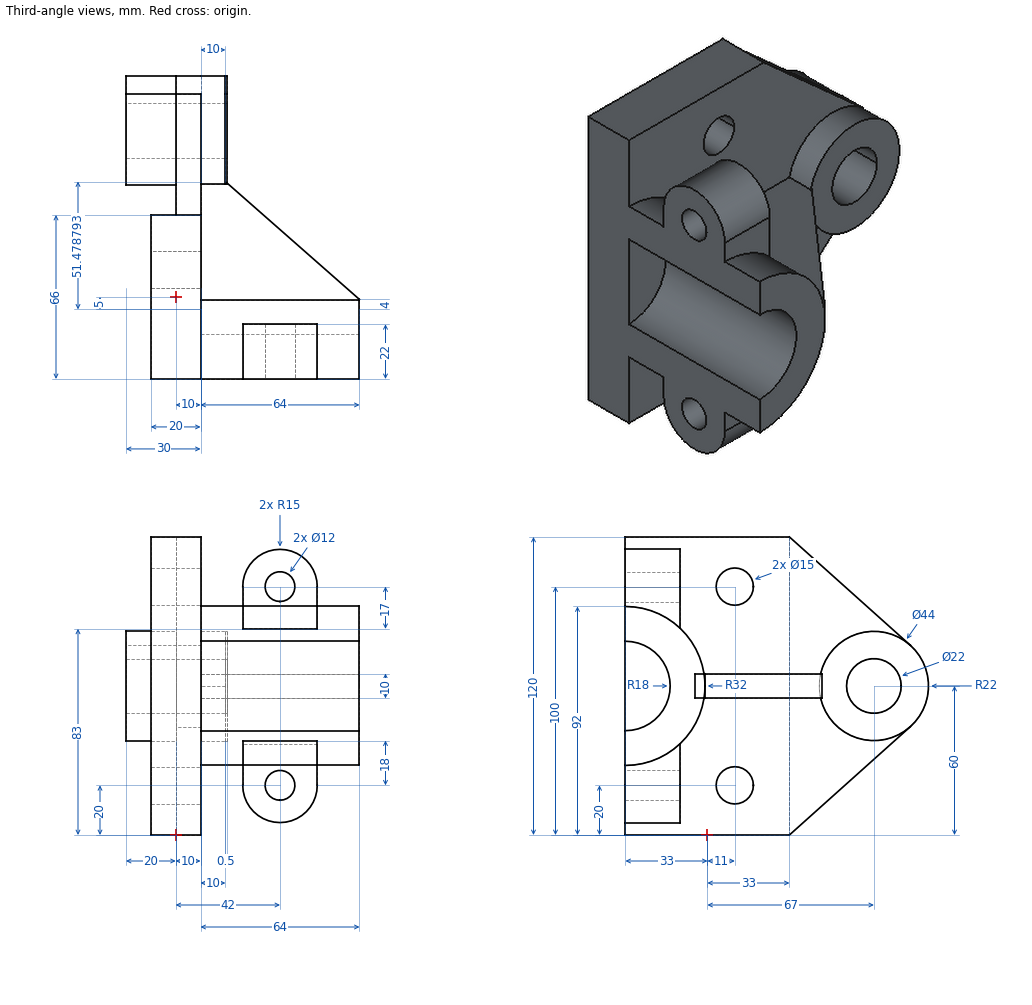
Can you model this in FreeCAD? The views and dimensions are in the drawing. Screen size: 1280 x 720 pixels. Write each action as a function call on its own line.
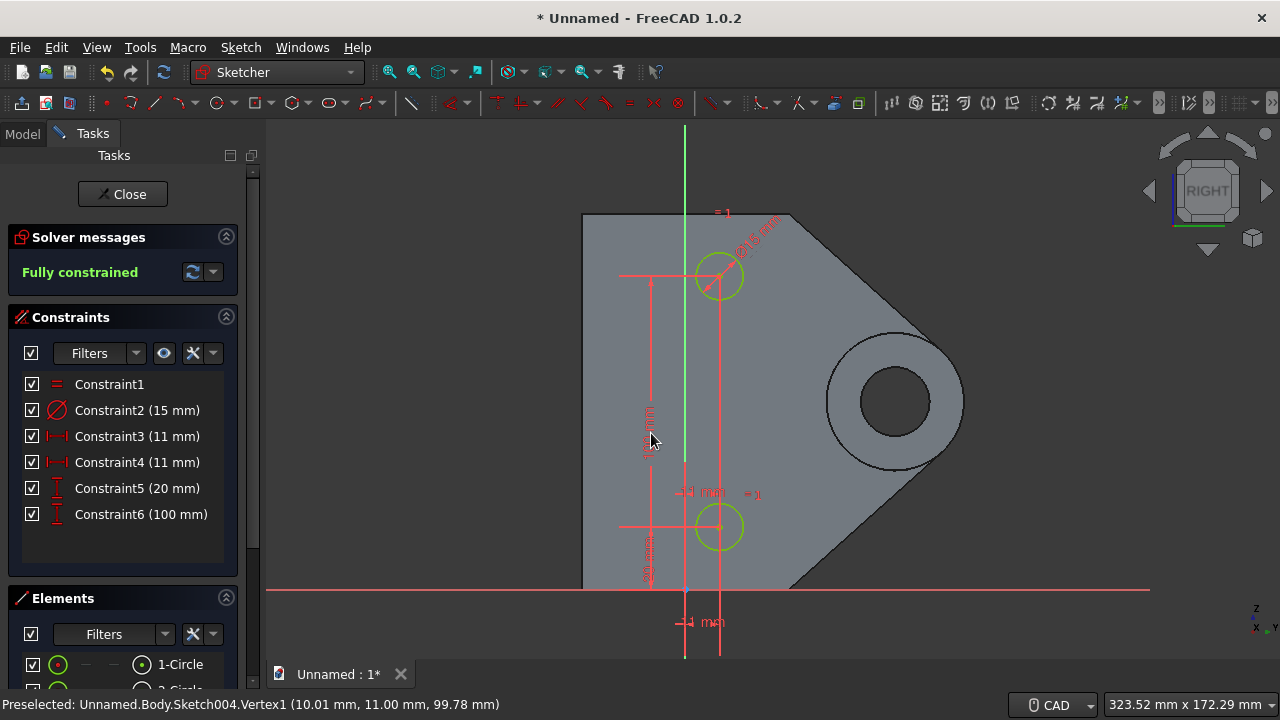
click(123, 194)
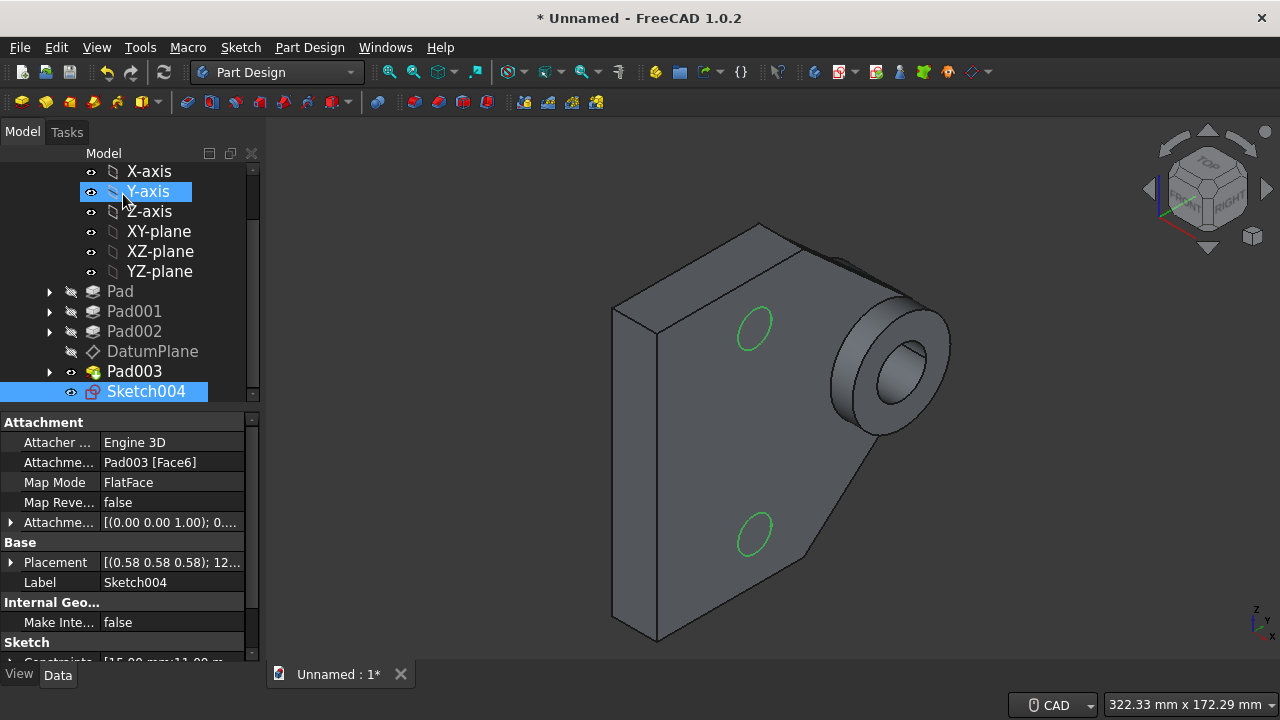
click(188, 102)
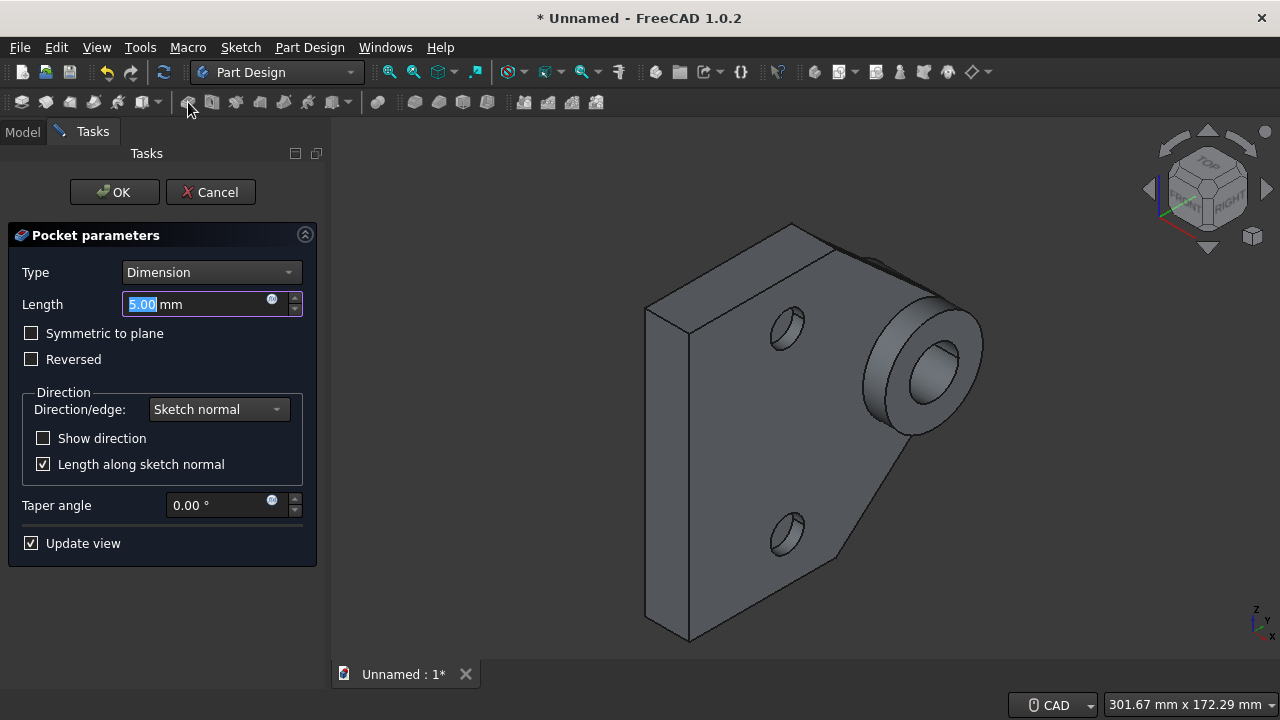
text(30)
key(Tab)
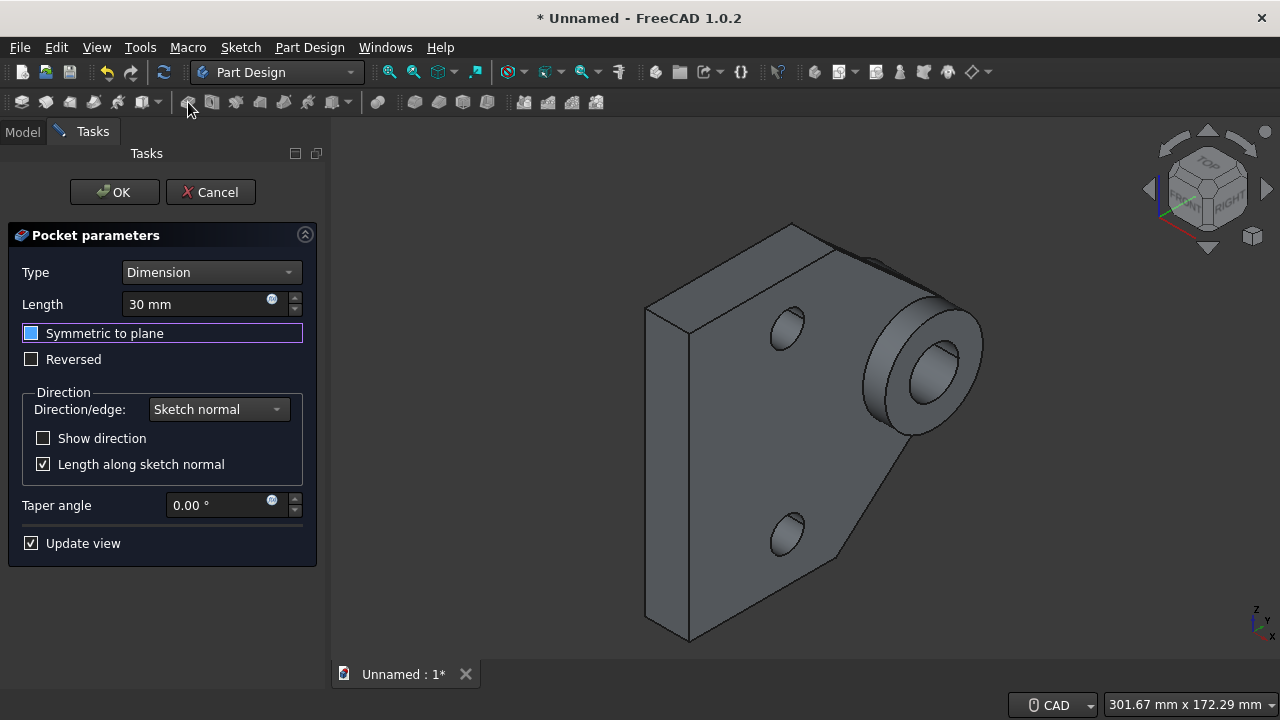
click(115, 192)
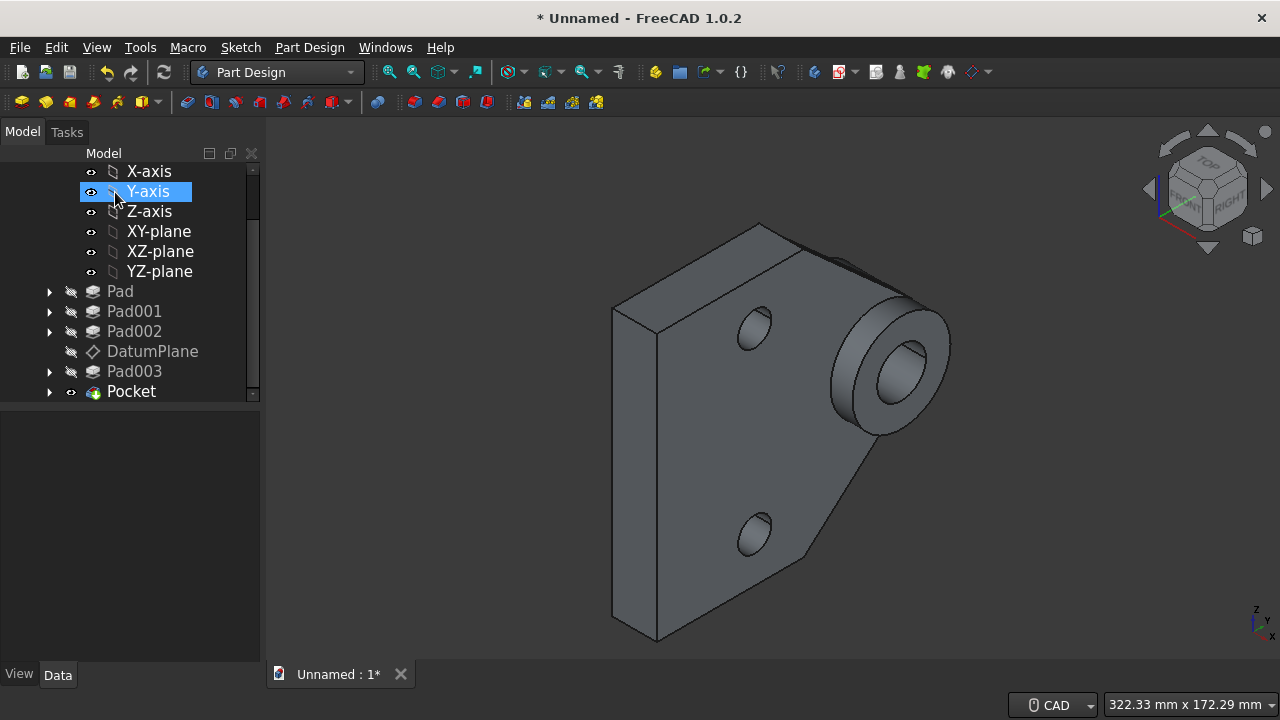
click(748, 434)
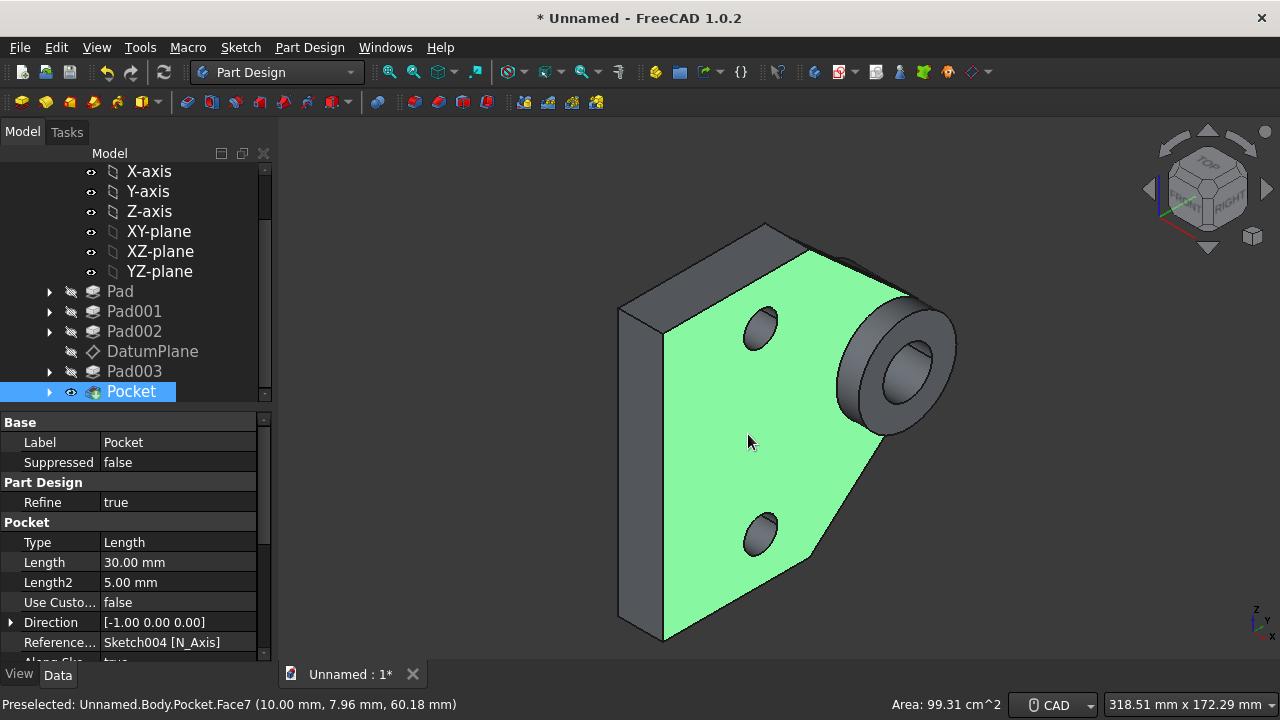
click(840, 72)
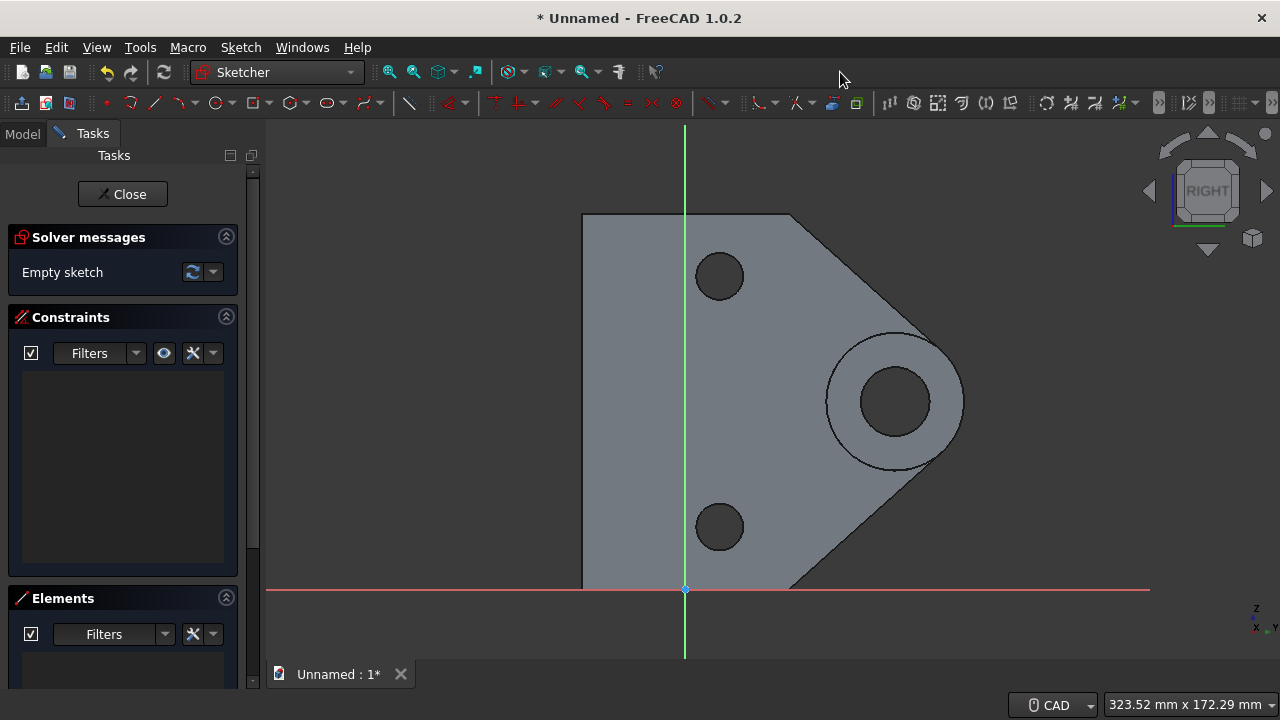
click(70, 104)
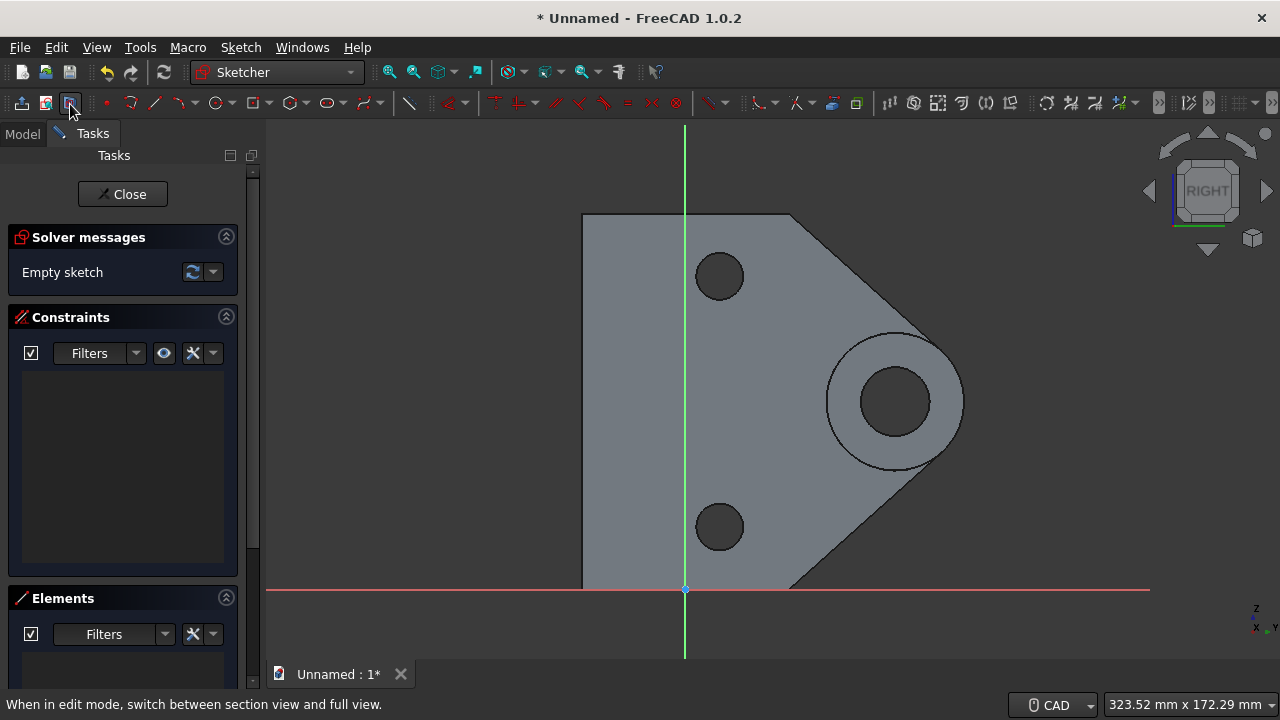
click(156, 104)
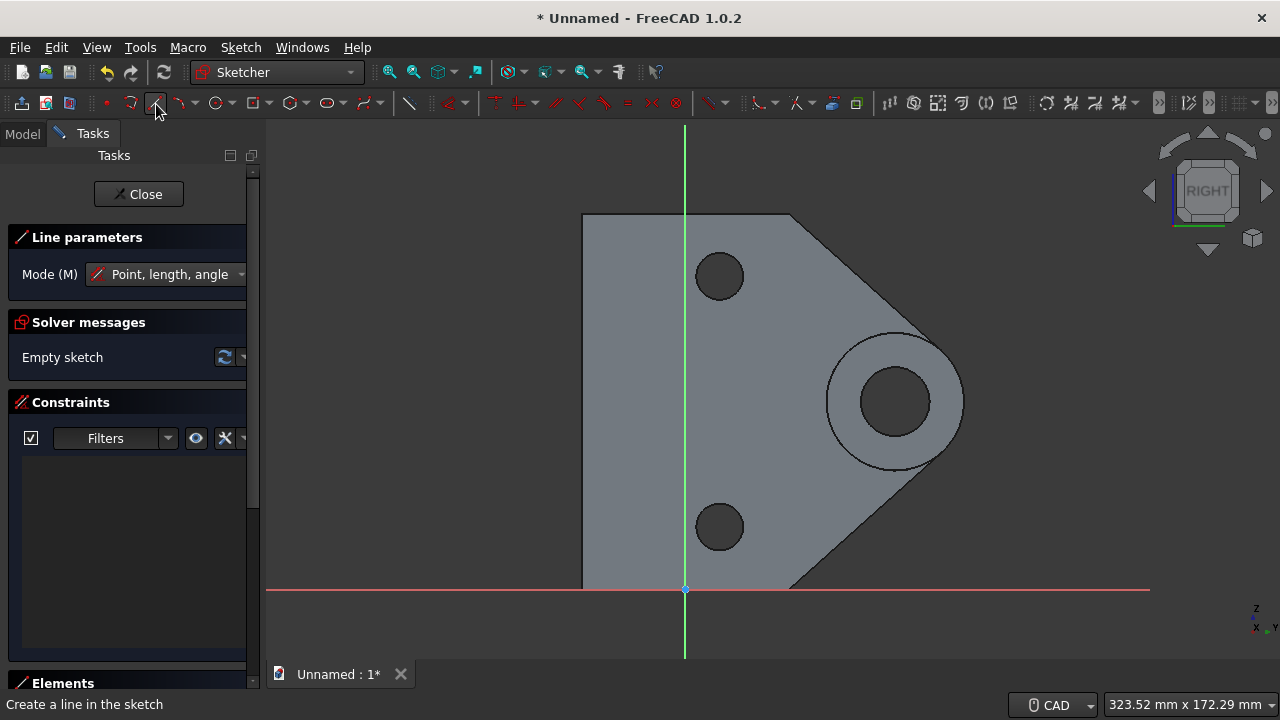
click(582, 301)
click(582, 345)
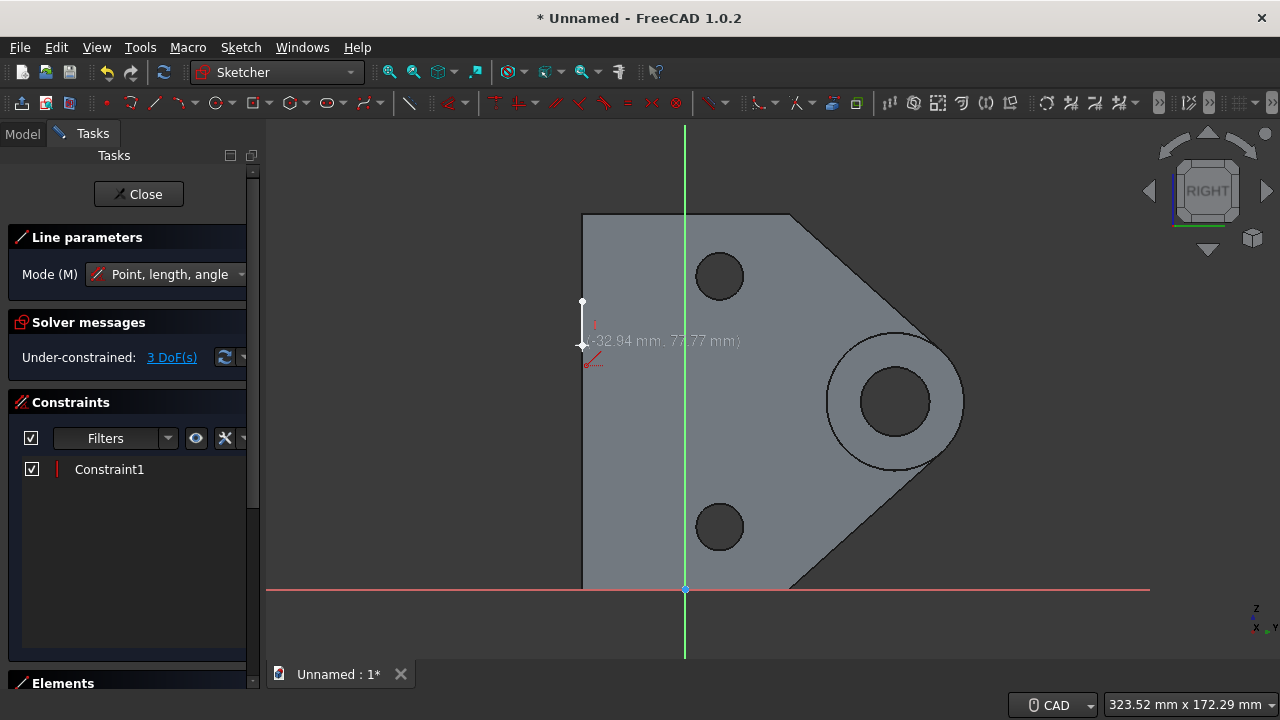
click(582, 458)
click(582, 502)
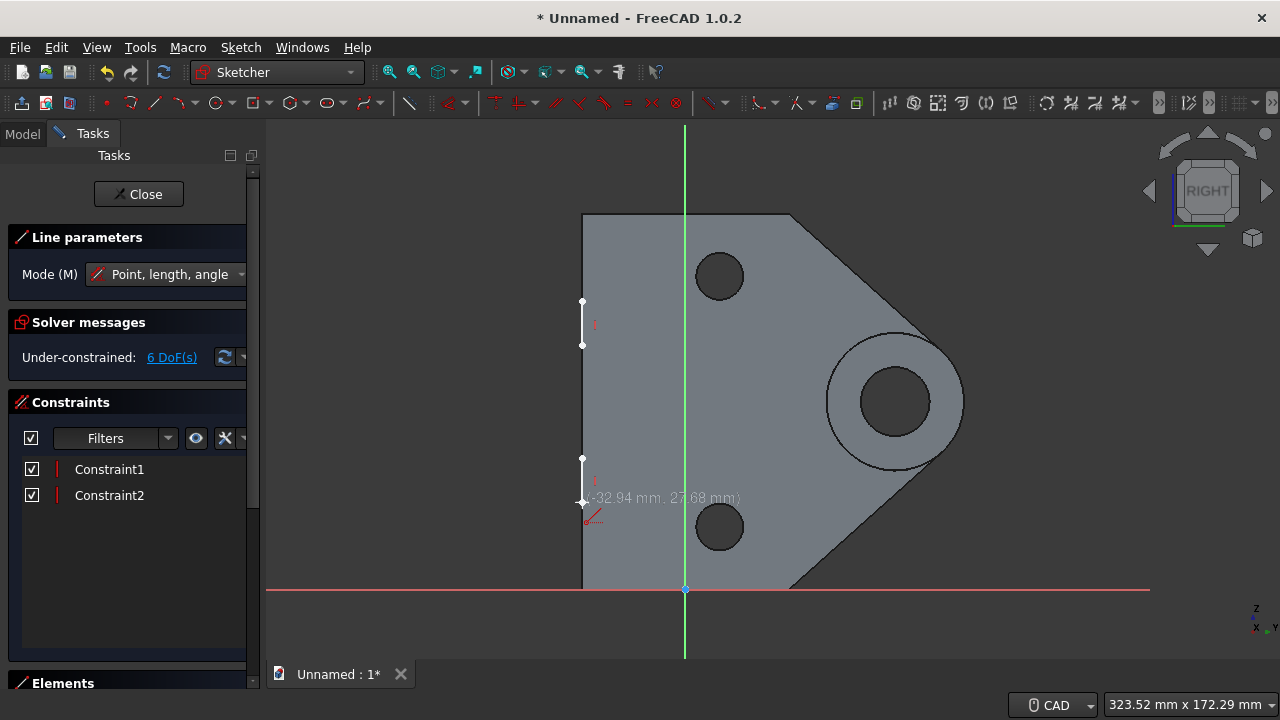
click(180, 104)